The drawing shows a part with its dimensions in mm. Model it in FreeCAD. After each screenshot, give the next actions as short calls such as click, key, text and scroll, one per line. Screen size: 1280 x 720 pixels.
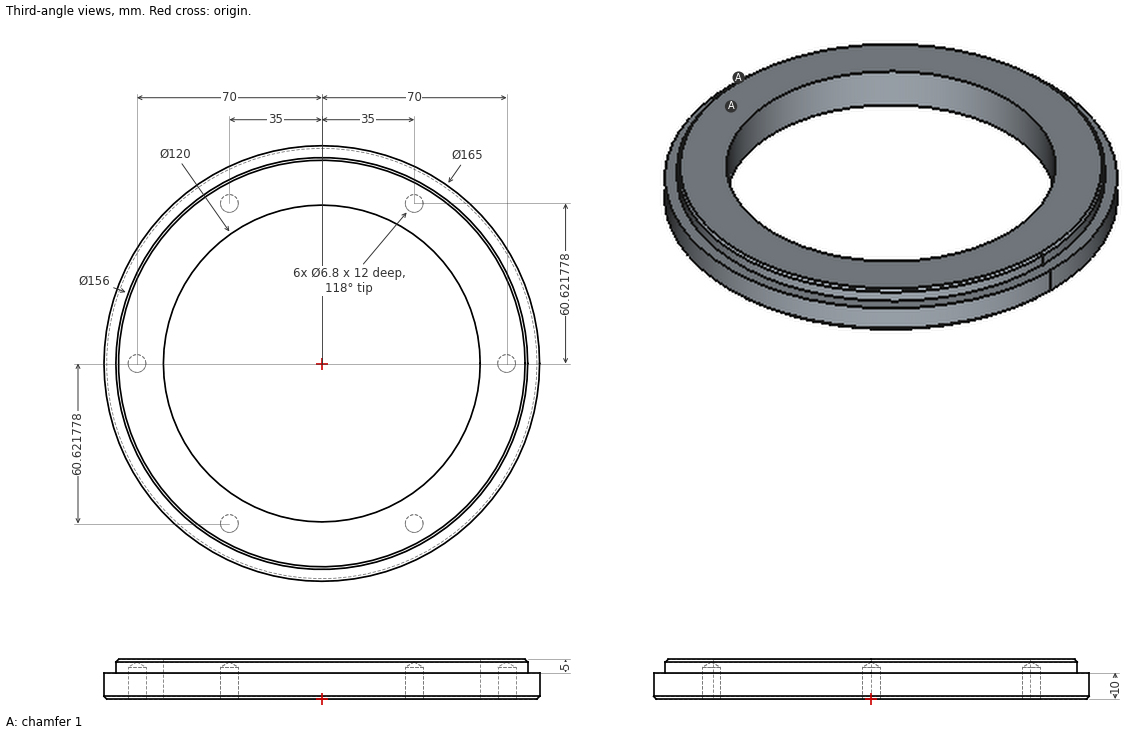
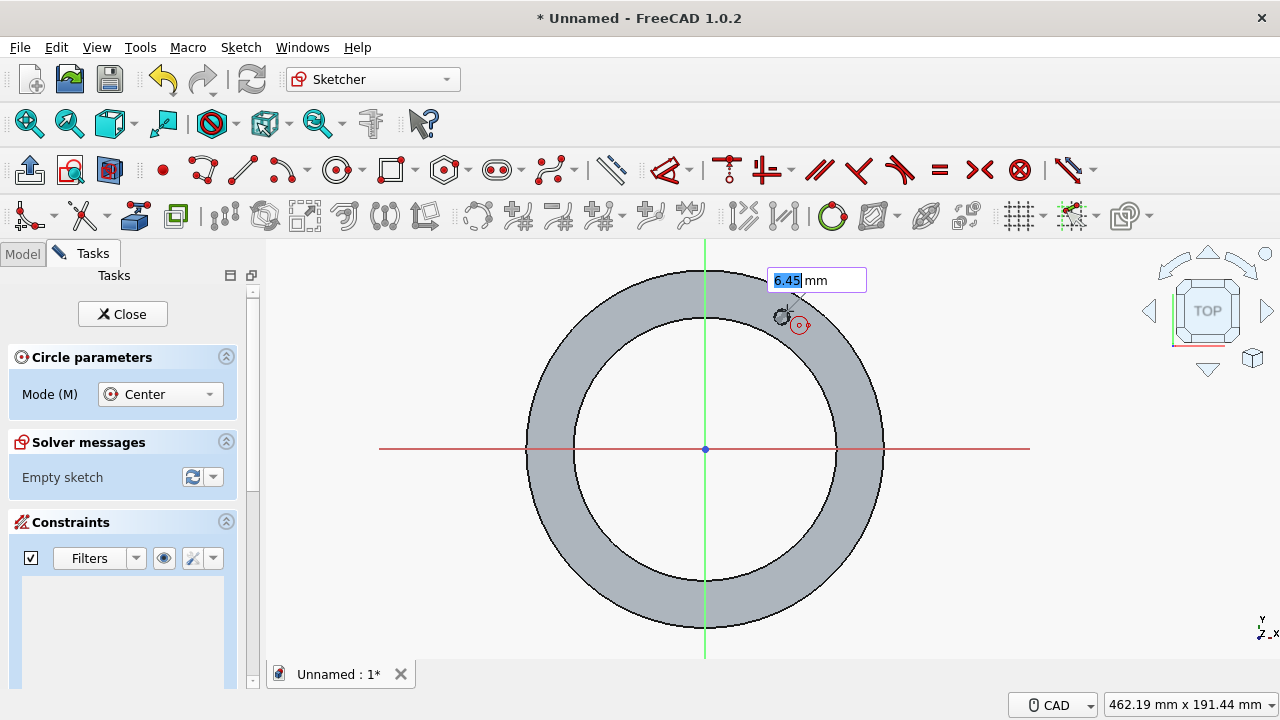
text(6.8)
key(Return)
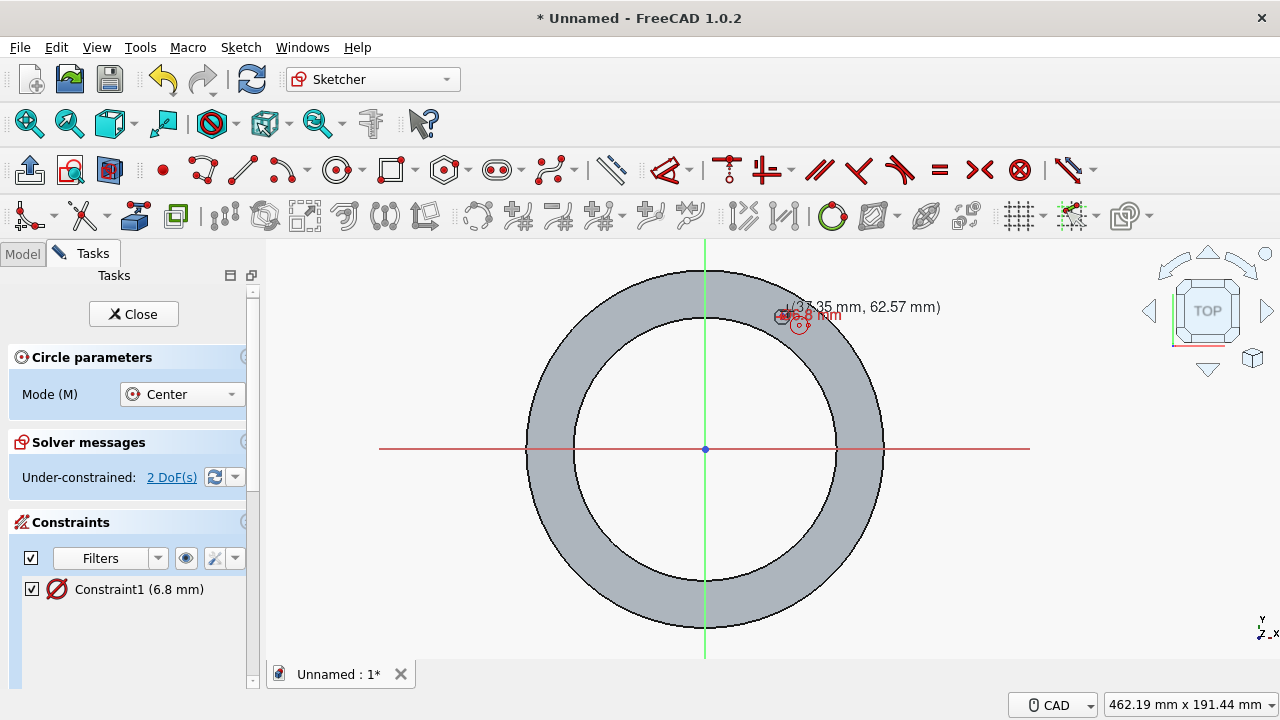
scroll(628, 316, up, 6)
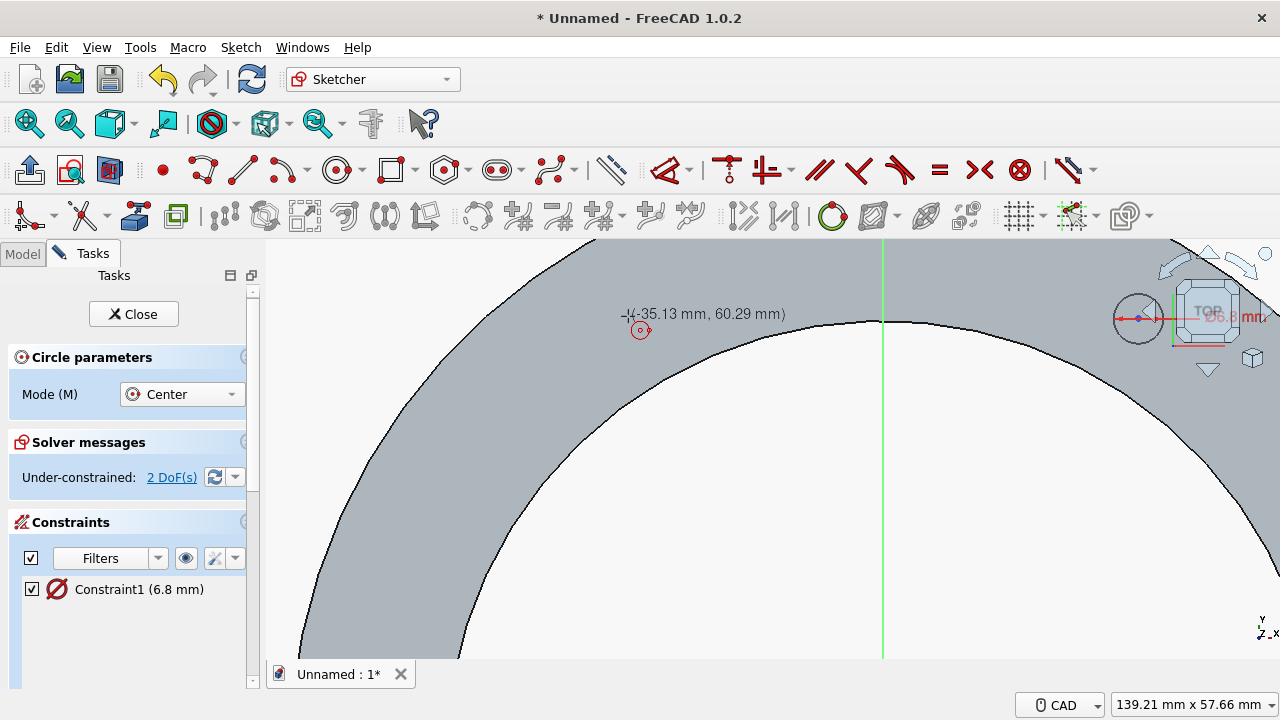
scroll(628, 316, down, 6)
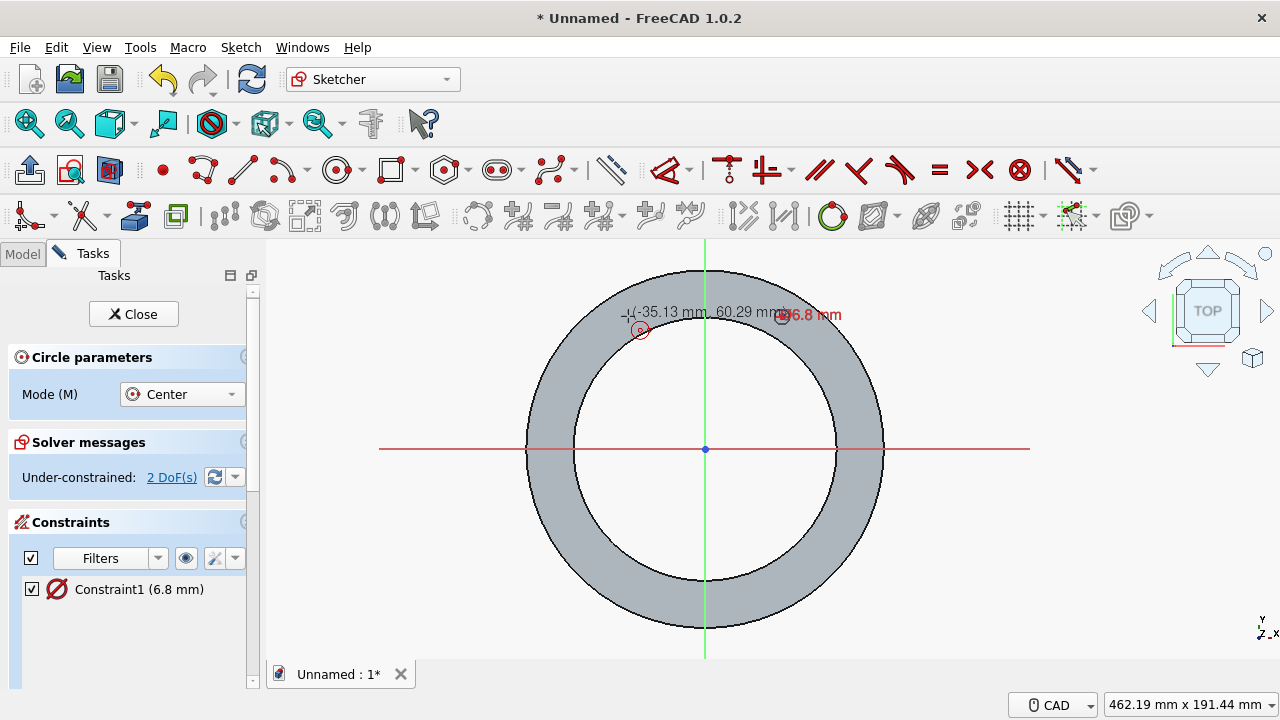
click(628, 316)
move(634, 311)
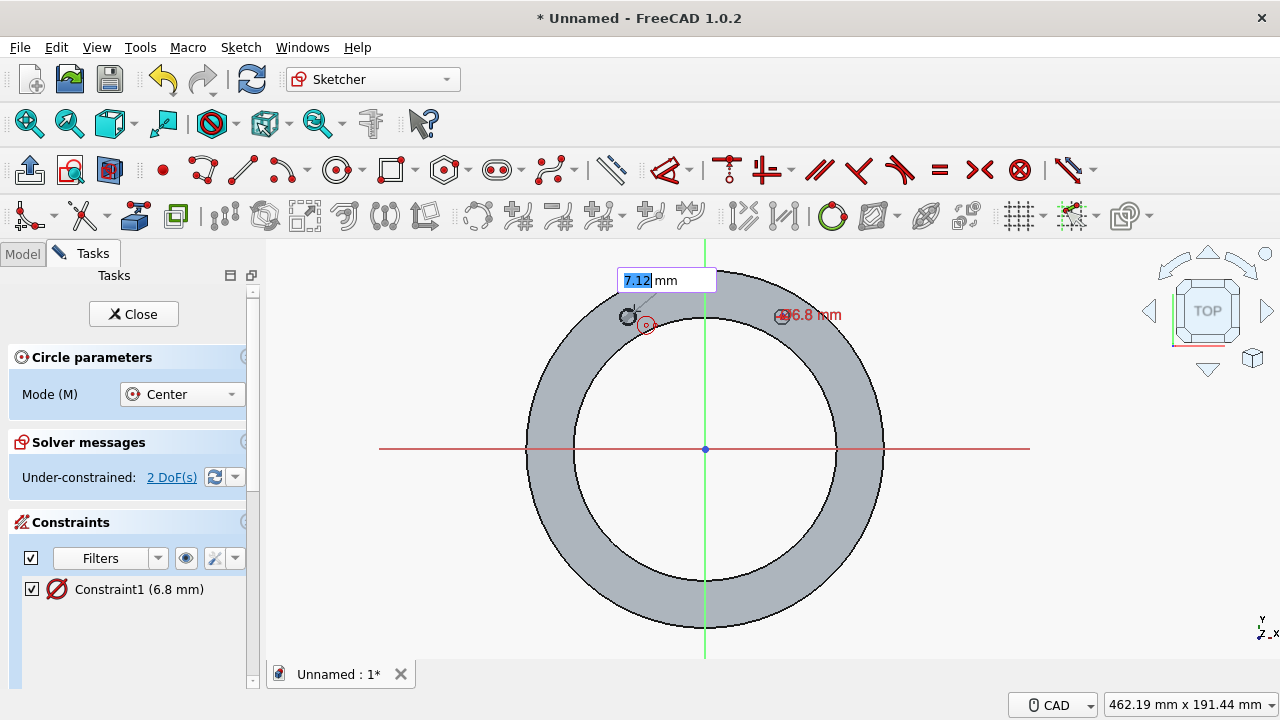
text(6.8)
key(Return)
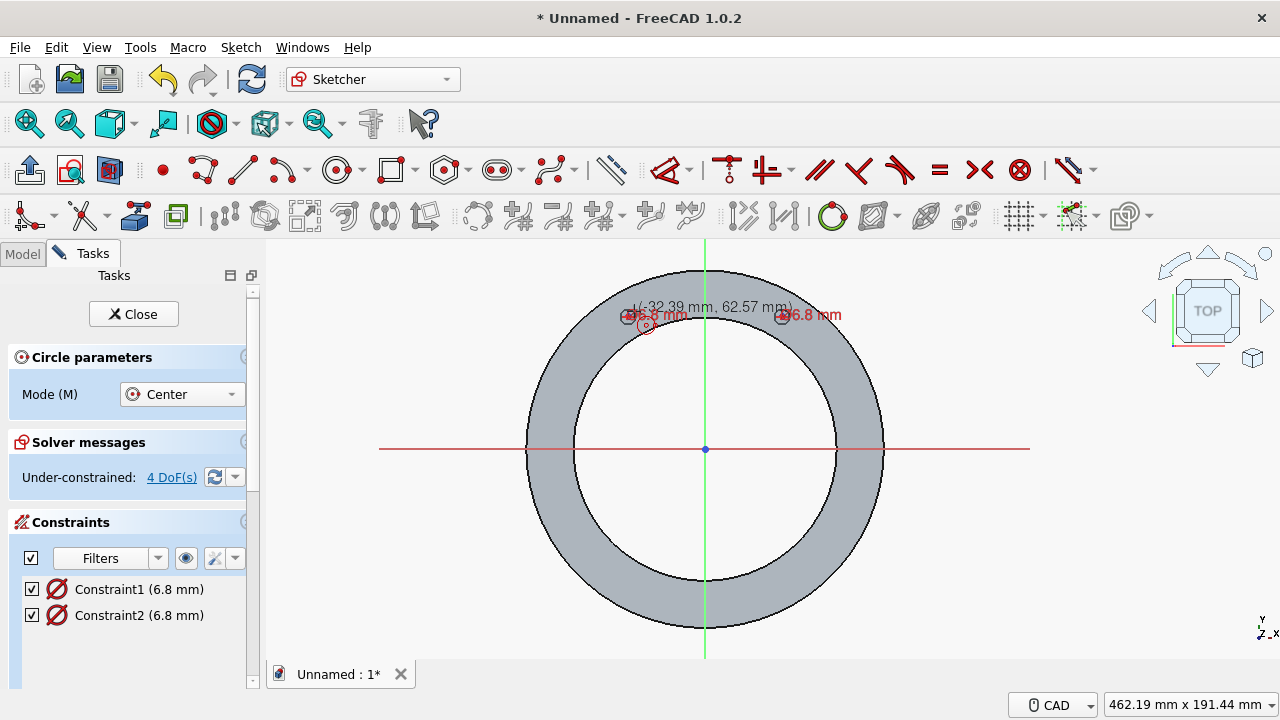
scroll(551, 449, up, 6)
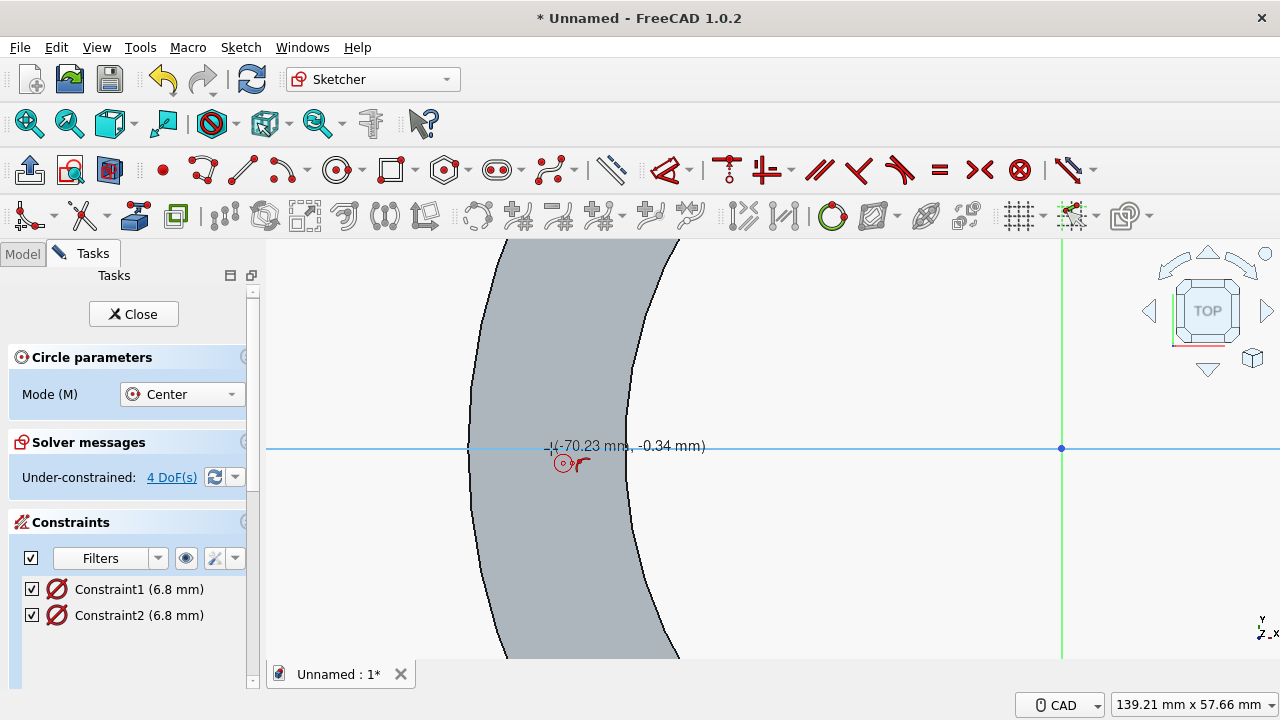
scroll(550, 449, down, 6)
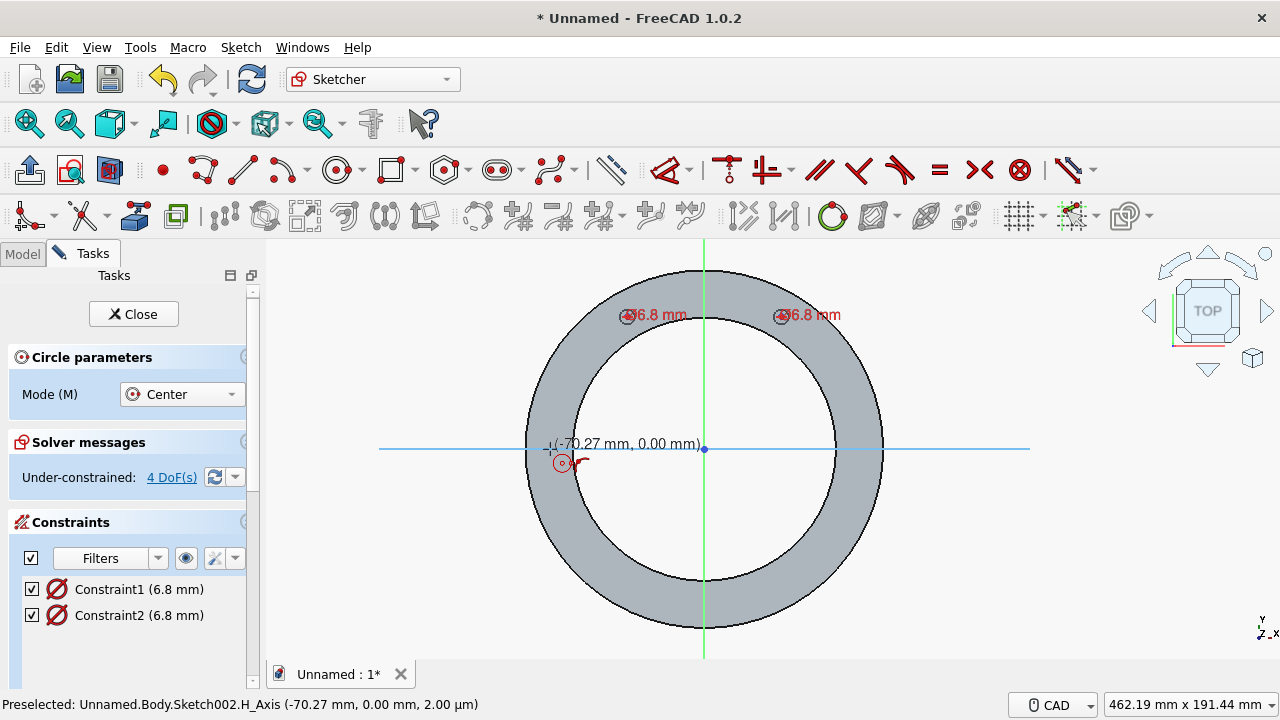
click(551, 449)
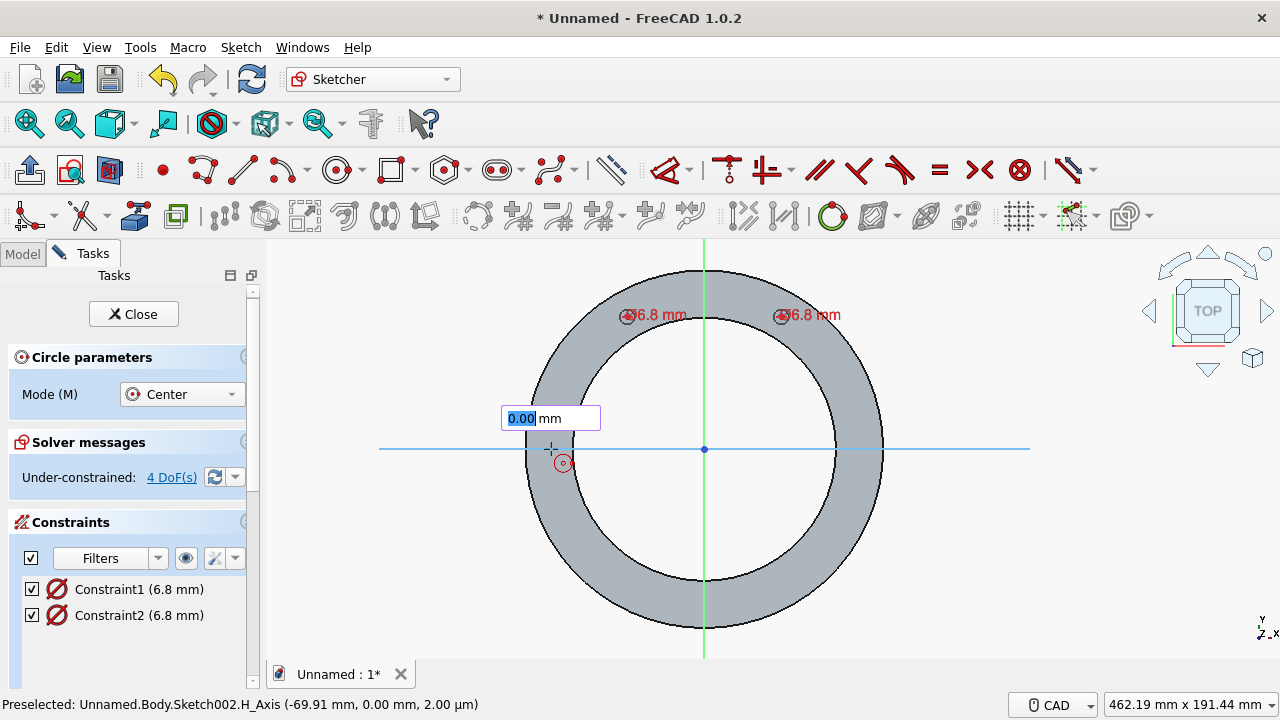
scroll(548, 456, up, 5)
move(548, 456)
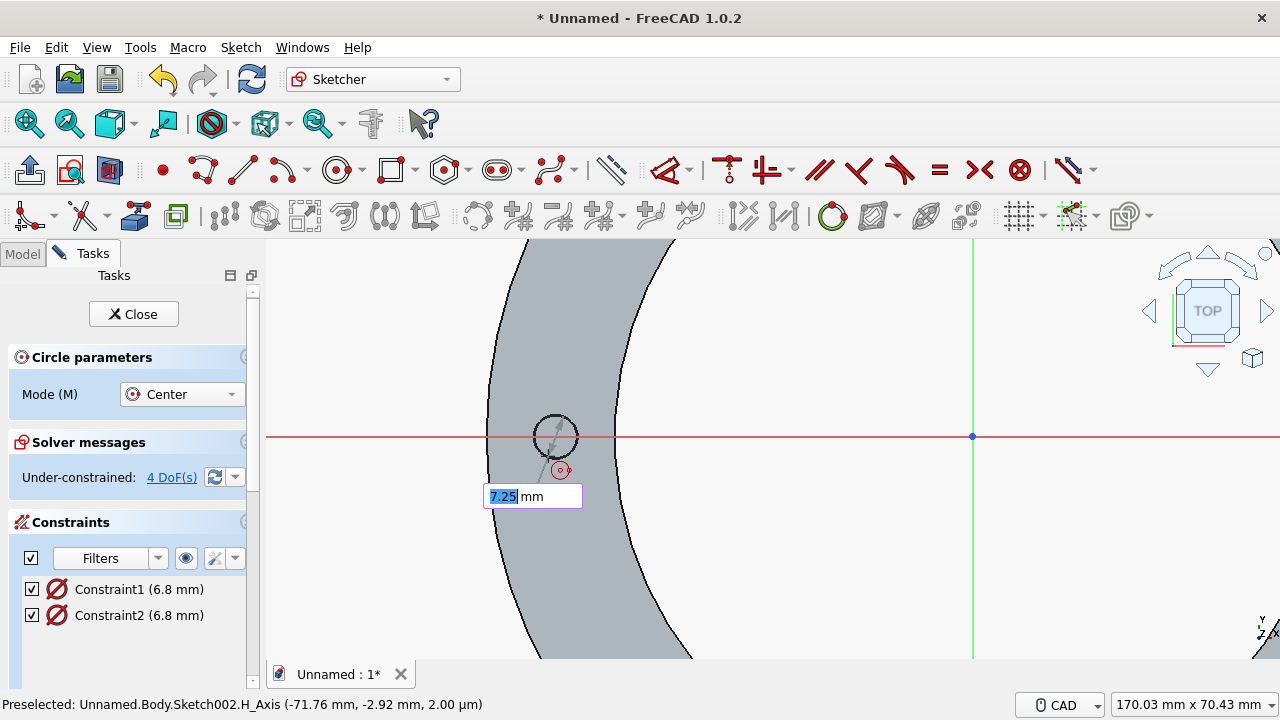
text(6.8)
key(Return)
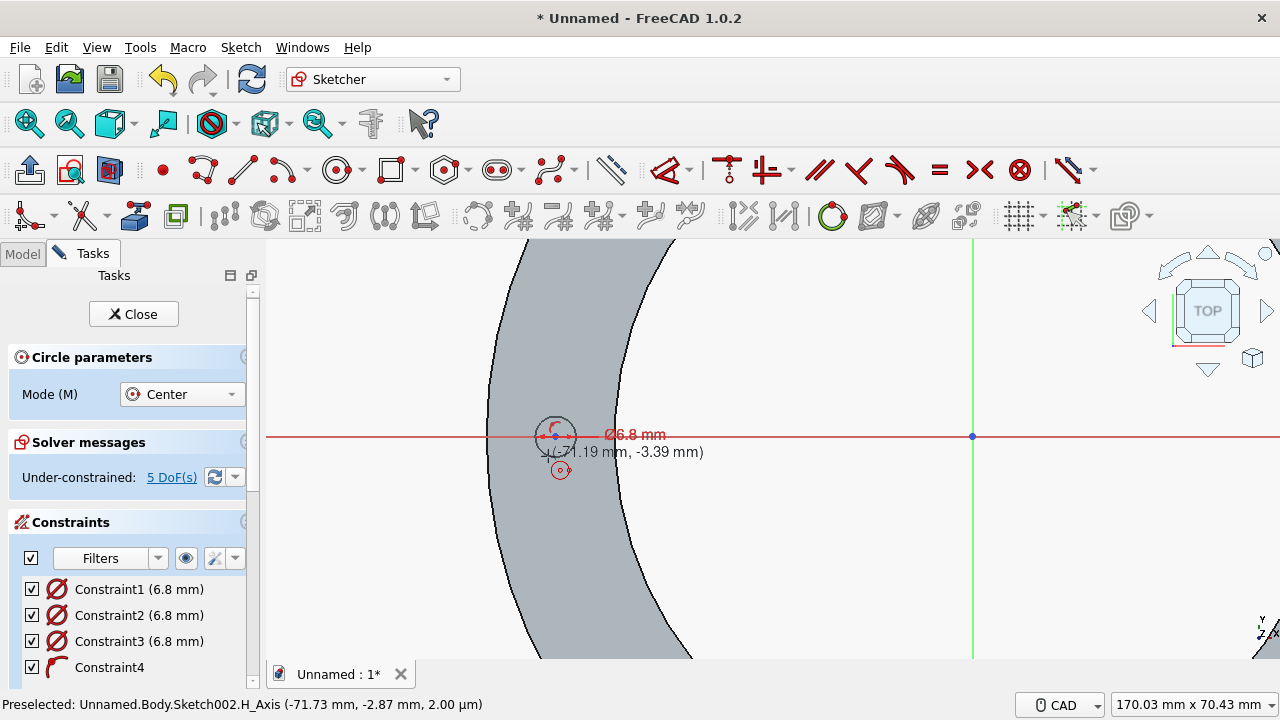
scroll(548, 456, down, 5)